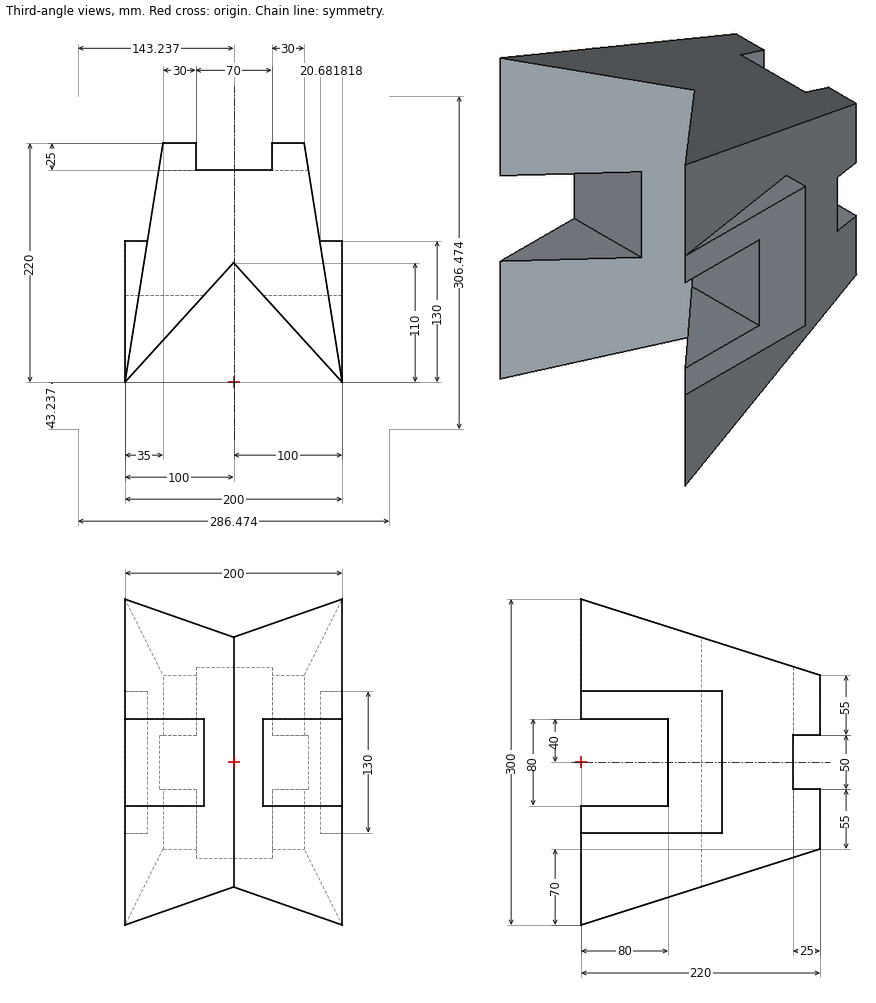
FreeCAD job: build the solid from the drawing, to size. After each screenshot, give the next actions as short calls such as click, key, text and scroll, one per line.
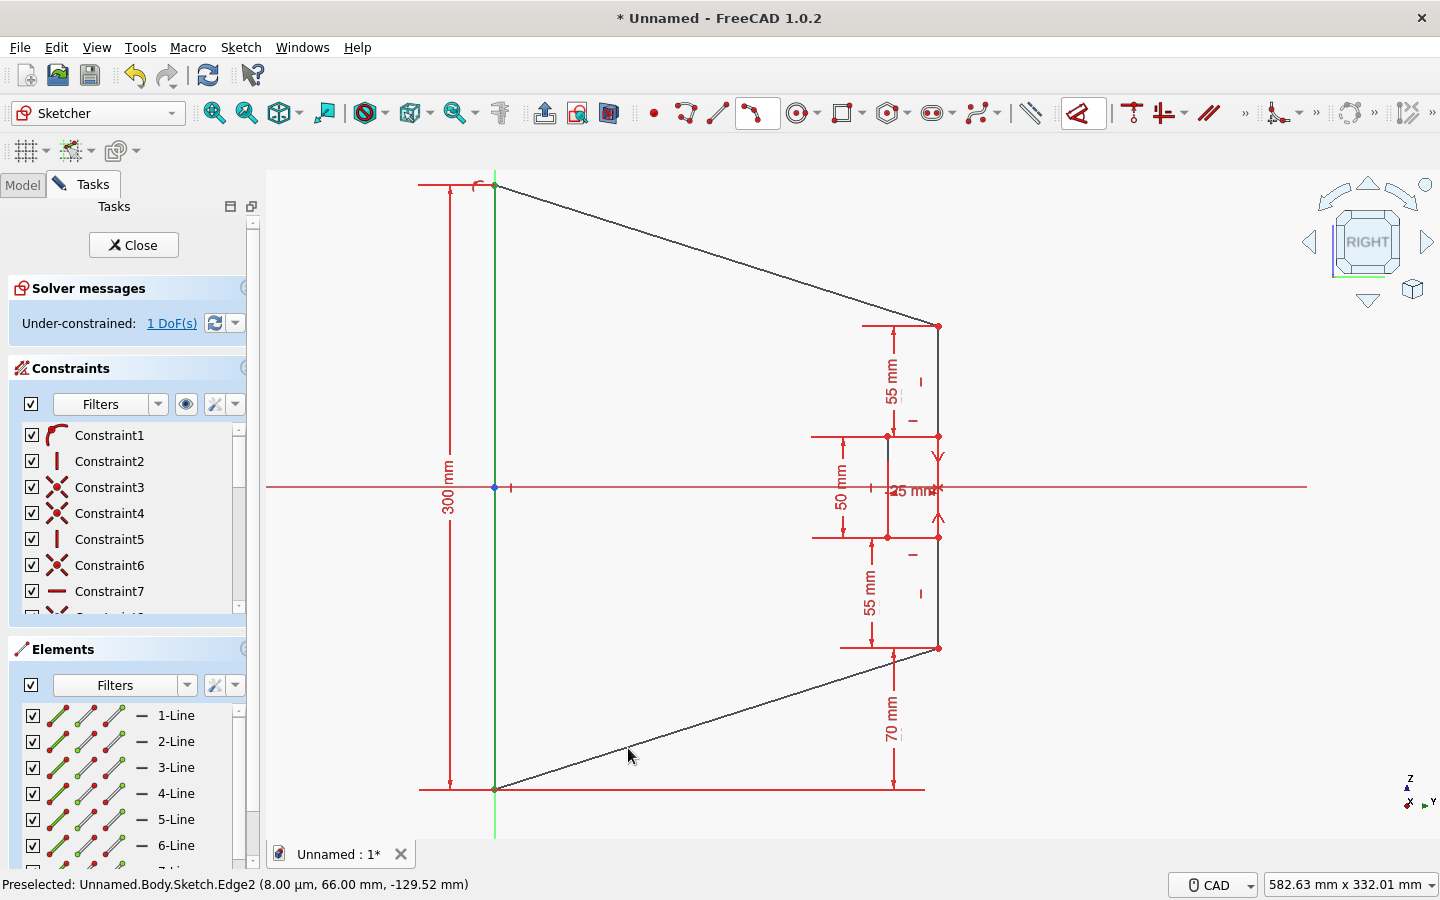
click(938, 648)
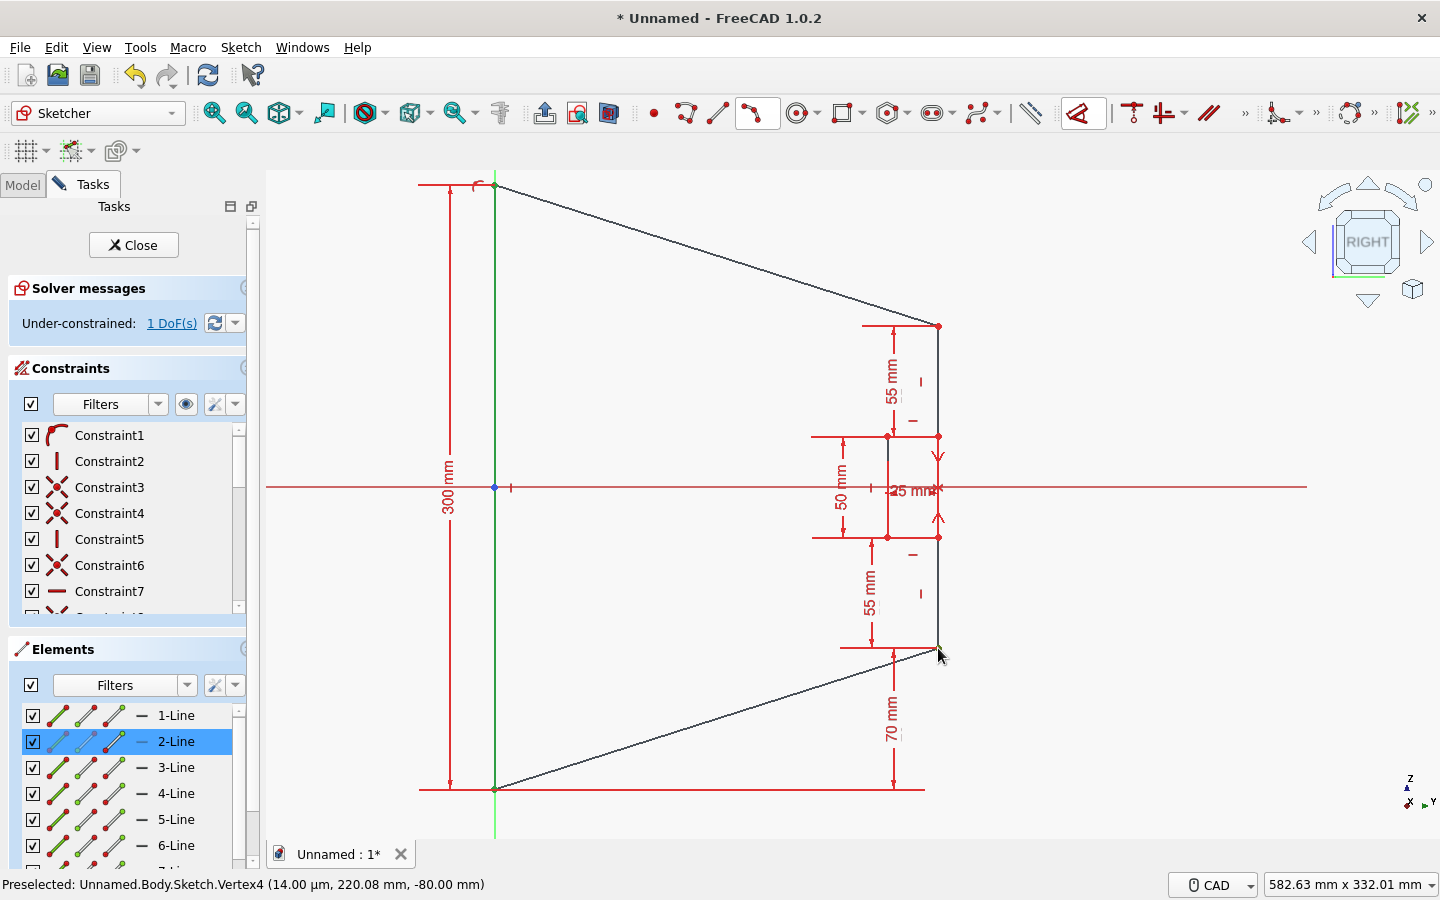
click(1100, 114)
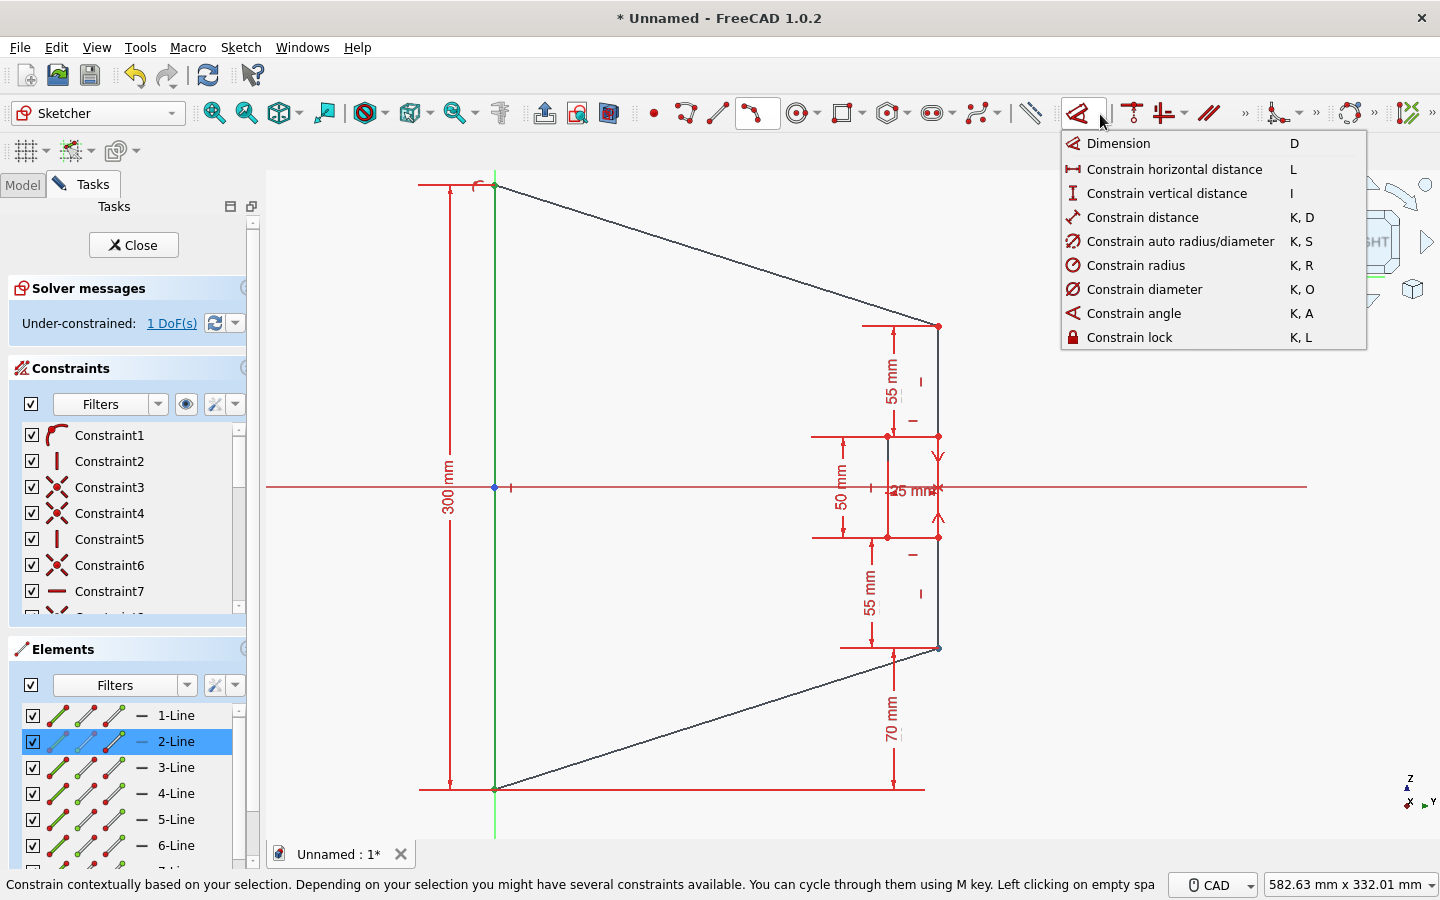
click(1214, 169)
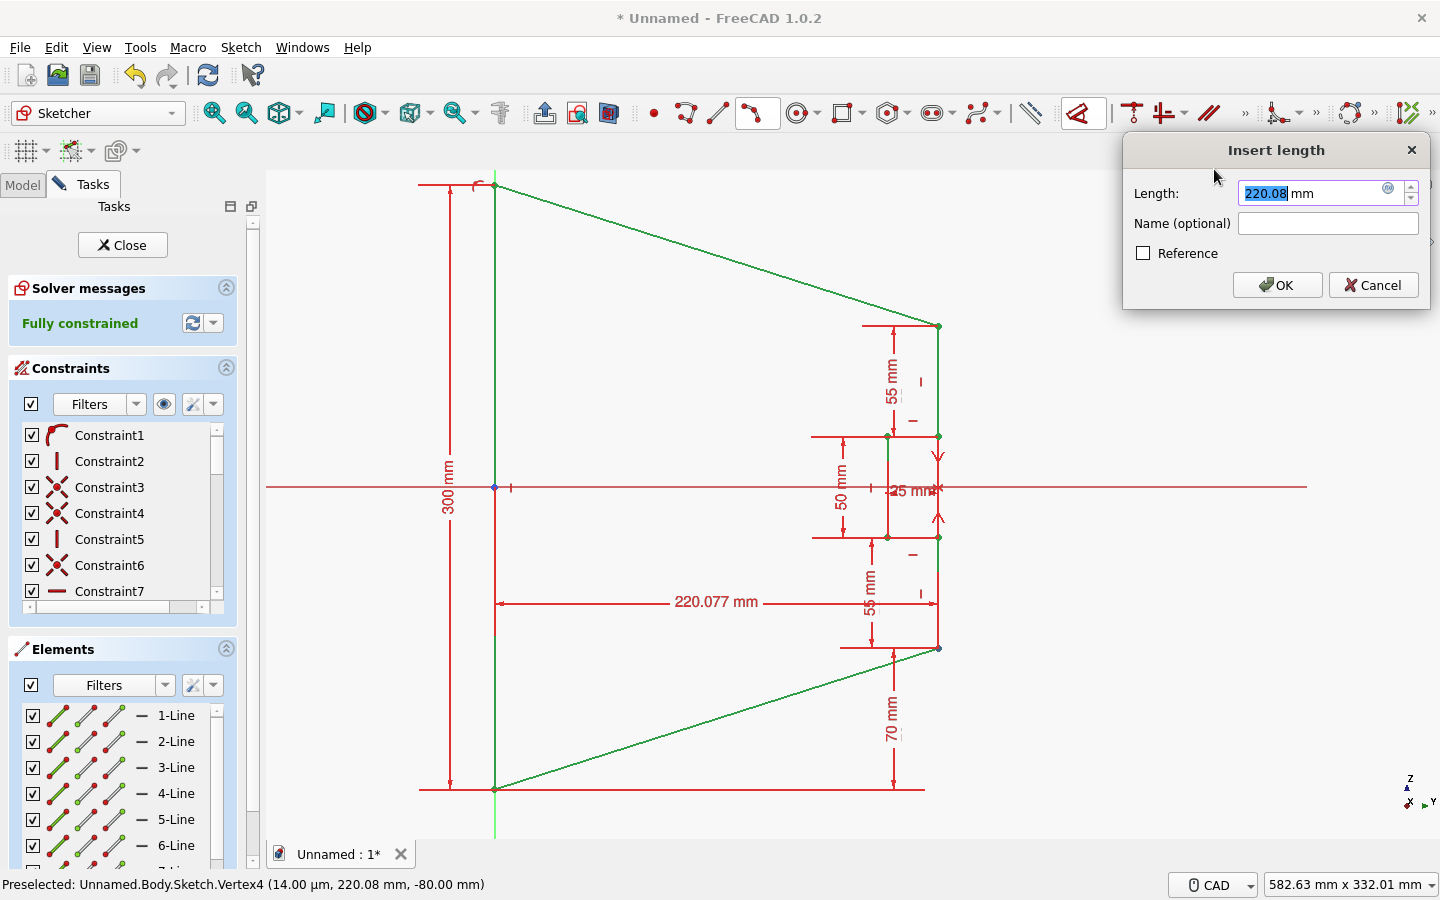
text(220)
key(Return)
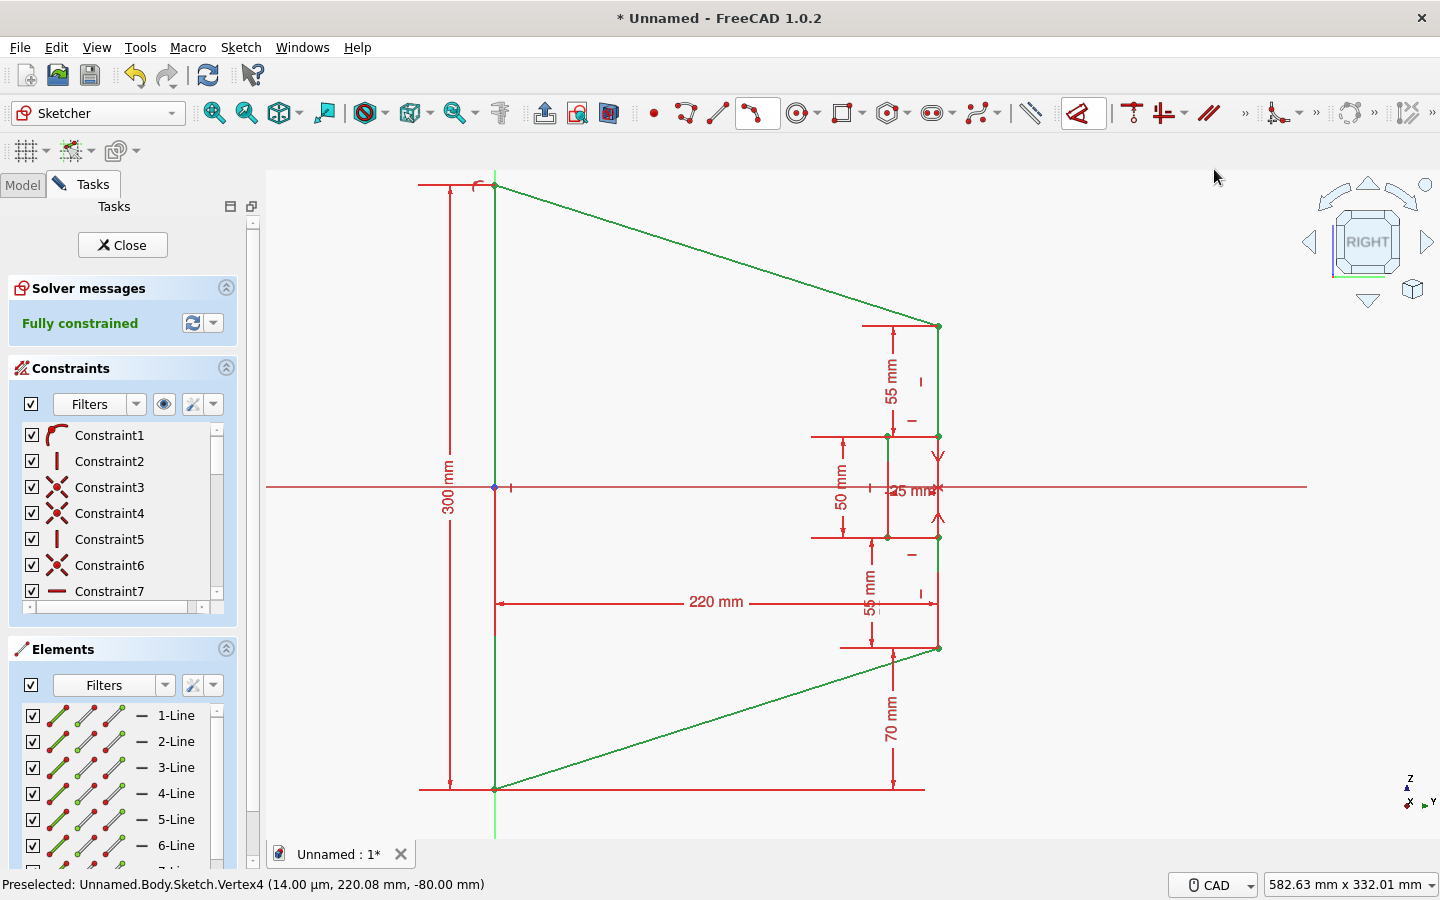
click(123, 245)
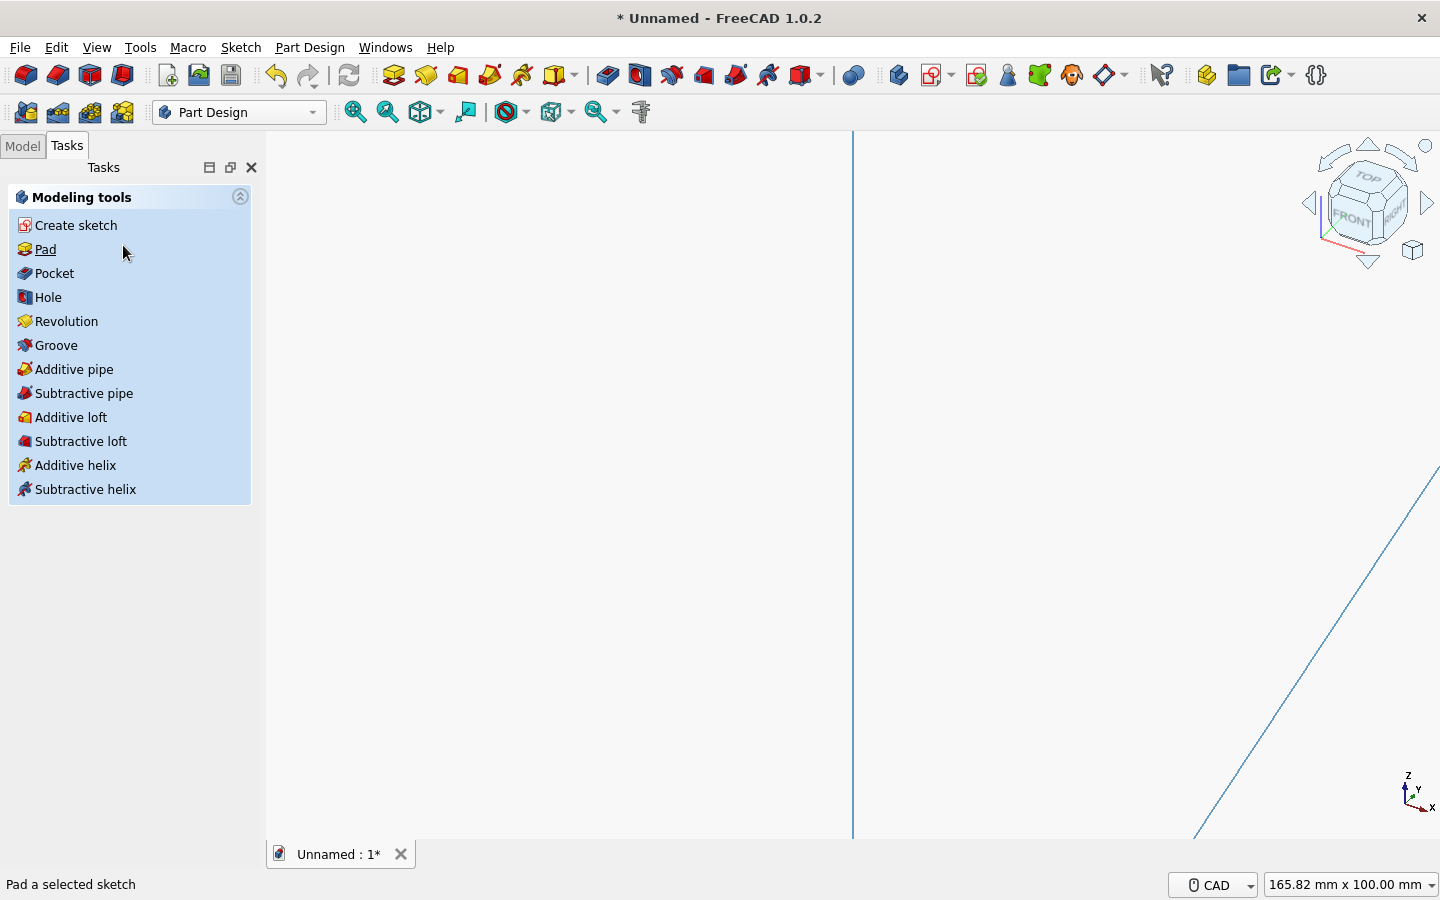
click(394, 76)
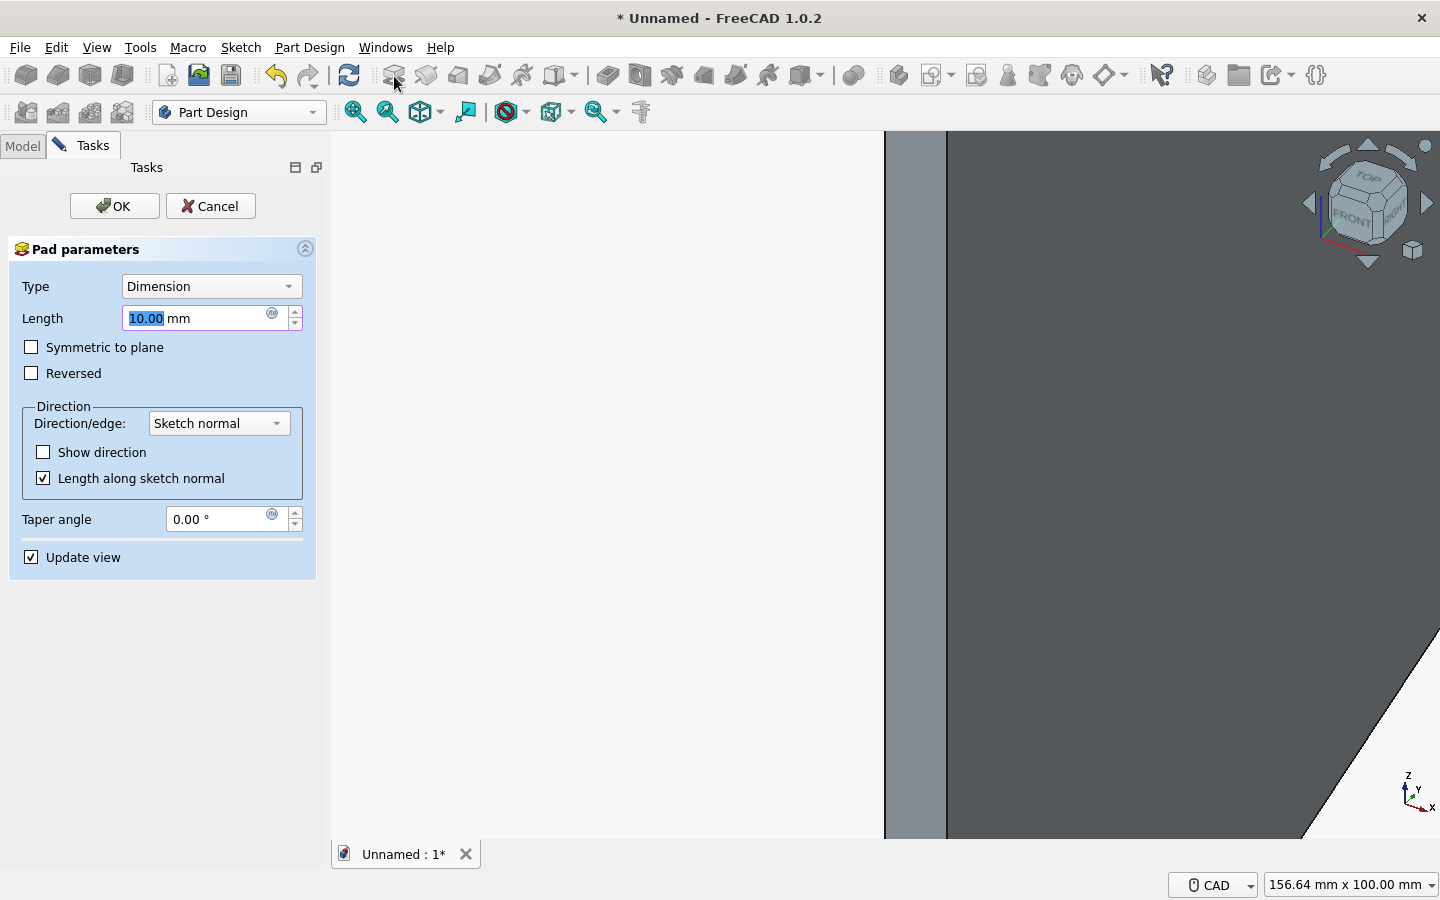
text(200)
key(Tab)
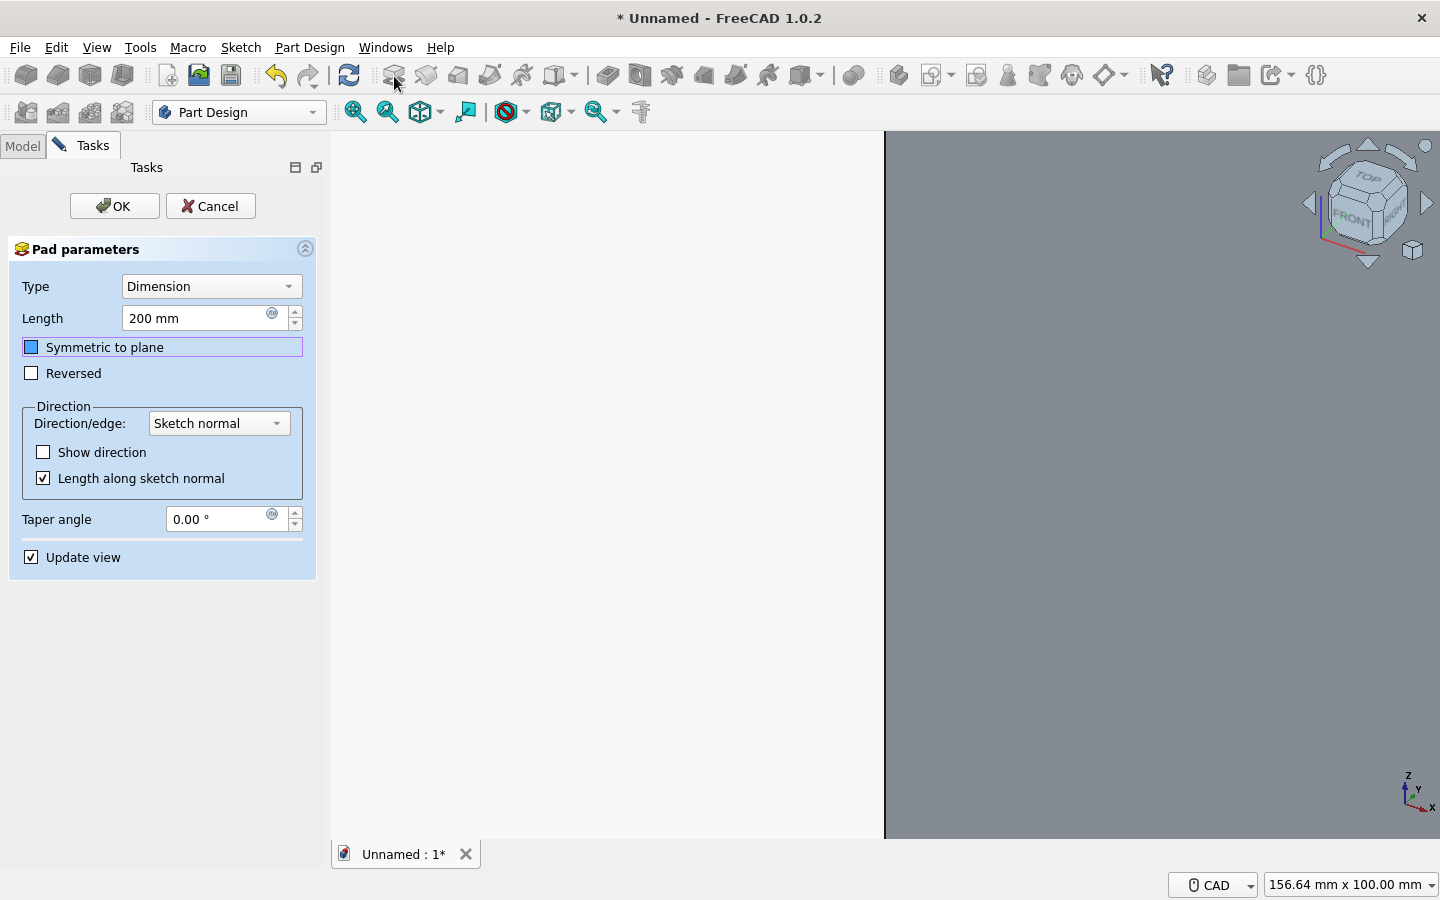
click(30, 347)